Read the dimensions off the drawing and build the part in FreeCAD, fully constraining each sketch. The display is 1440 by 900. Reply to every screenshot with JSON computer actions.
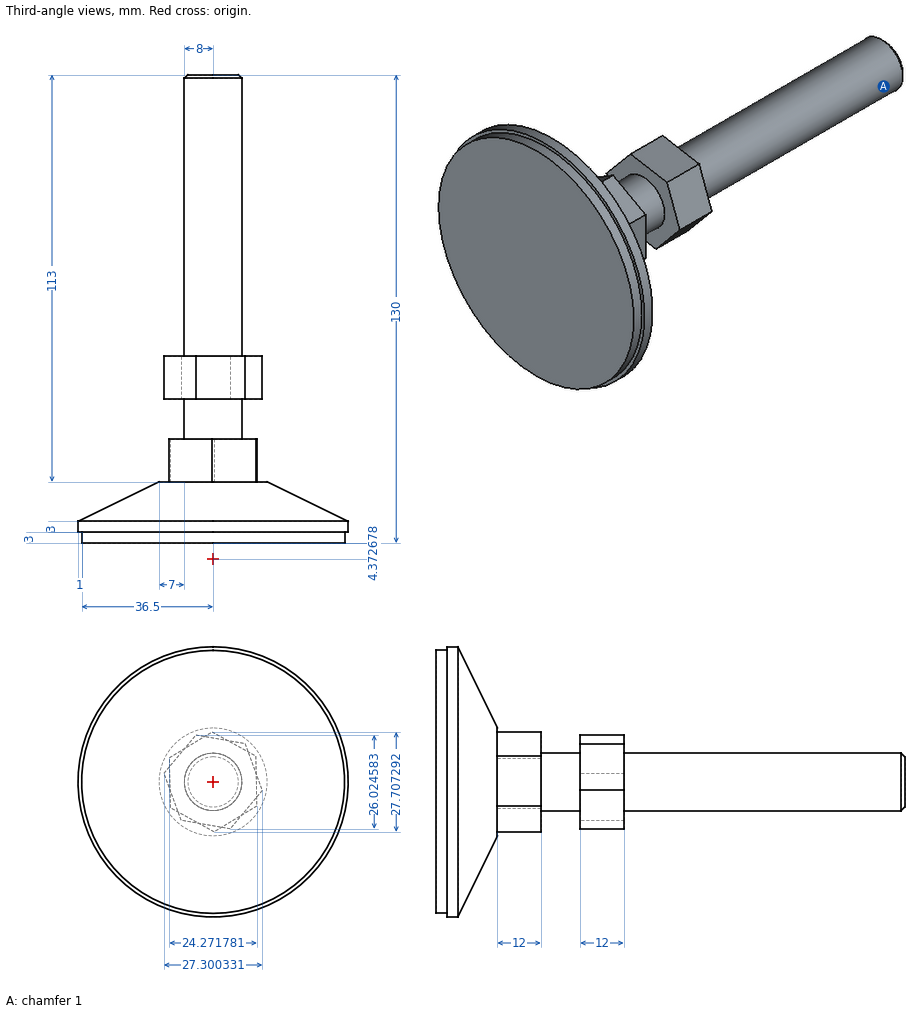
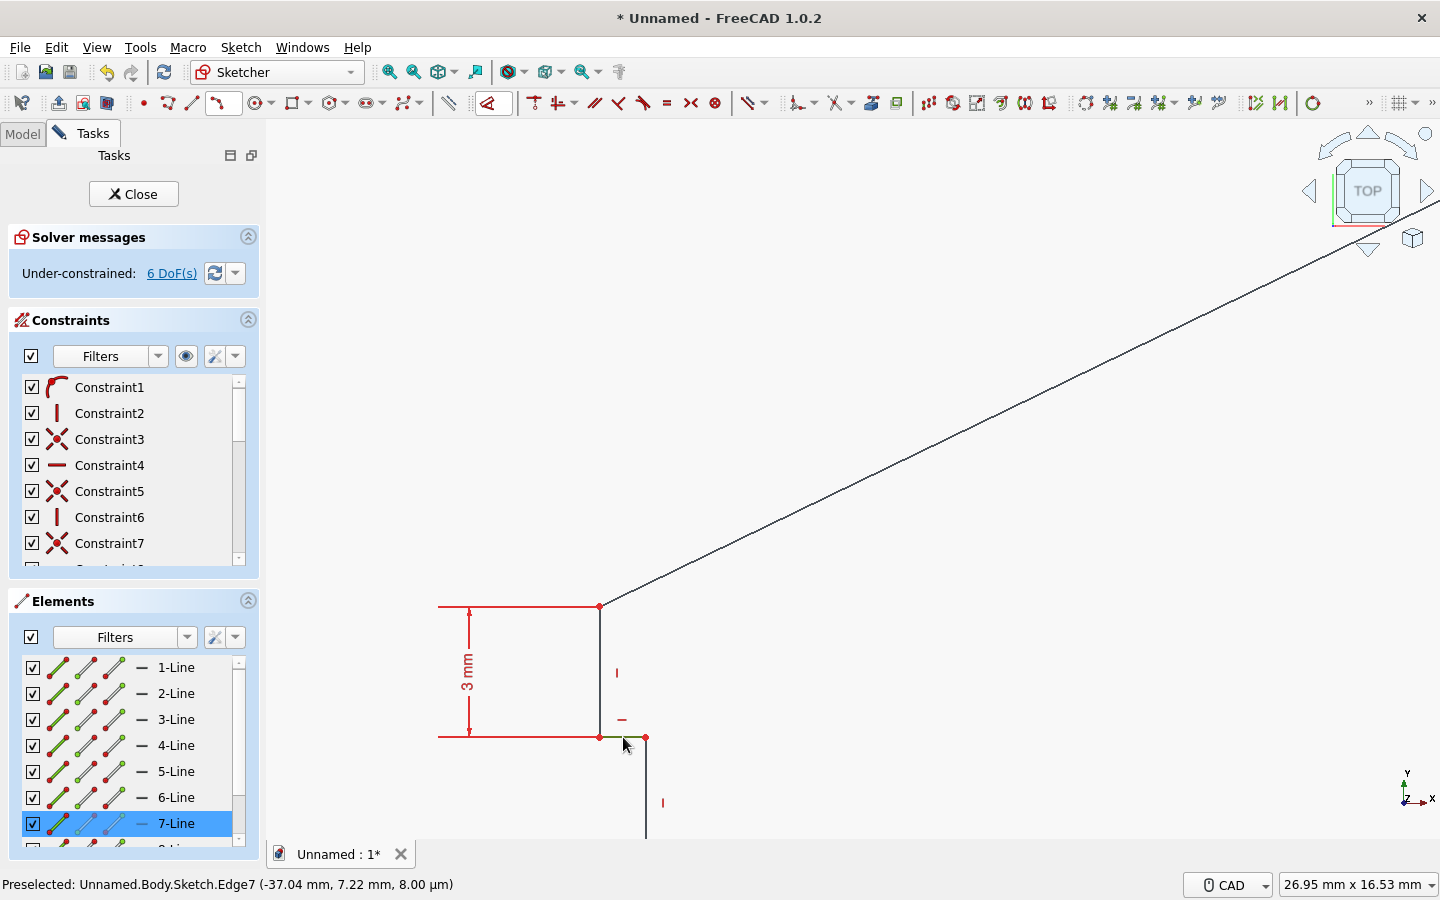
{"action": "left_click", "coordinate": [506, 104]}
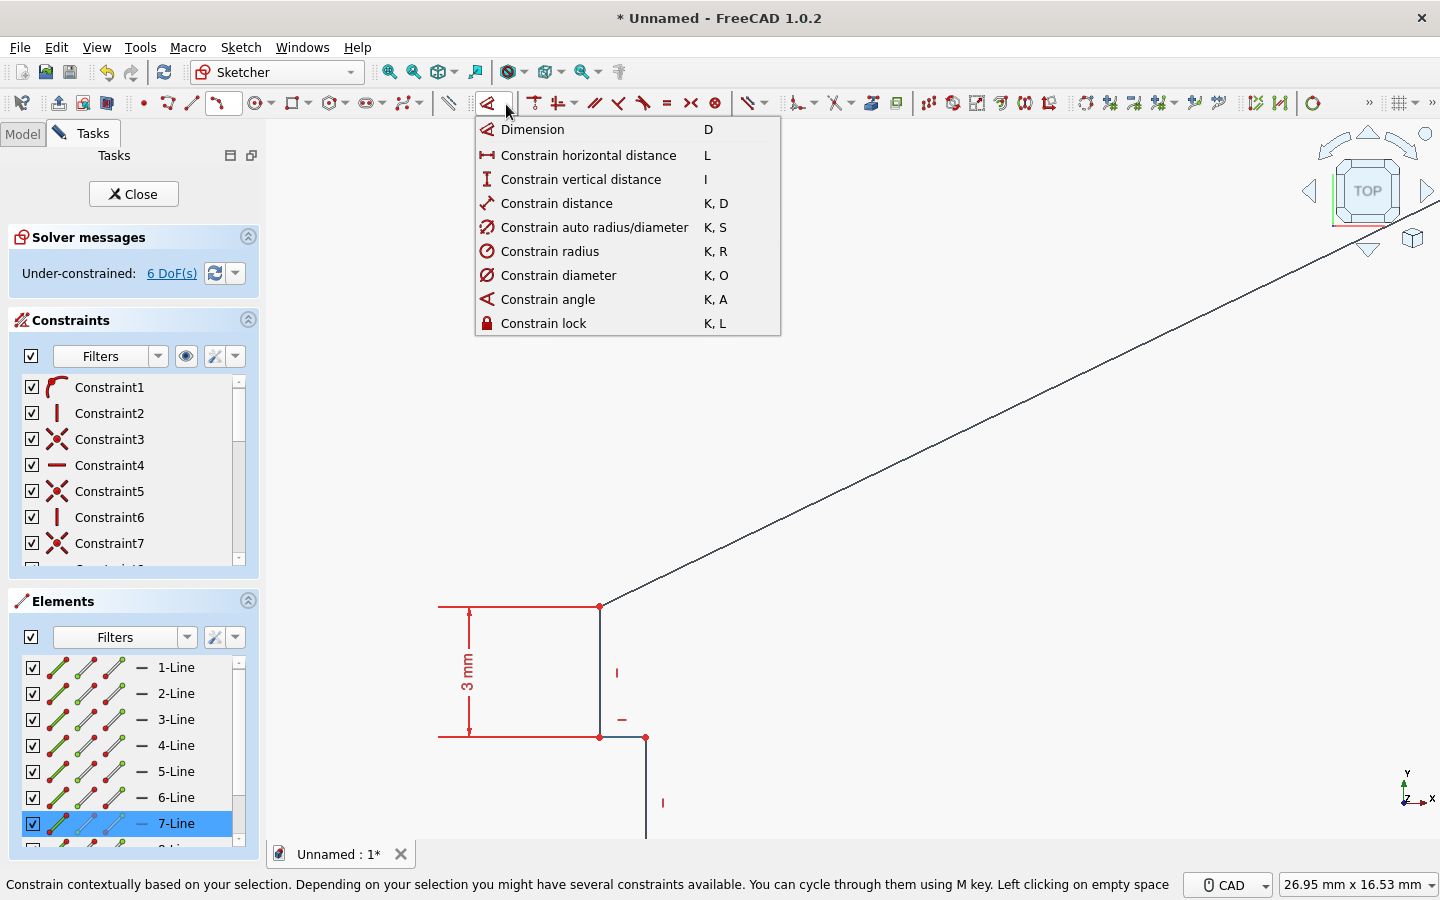
{"action": "left_click", "coordinate": [628, 155]}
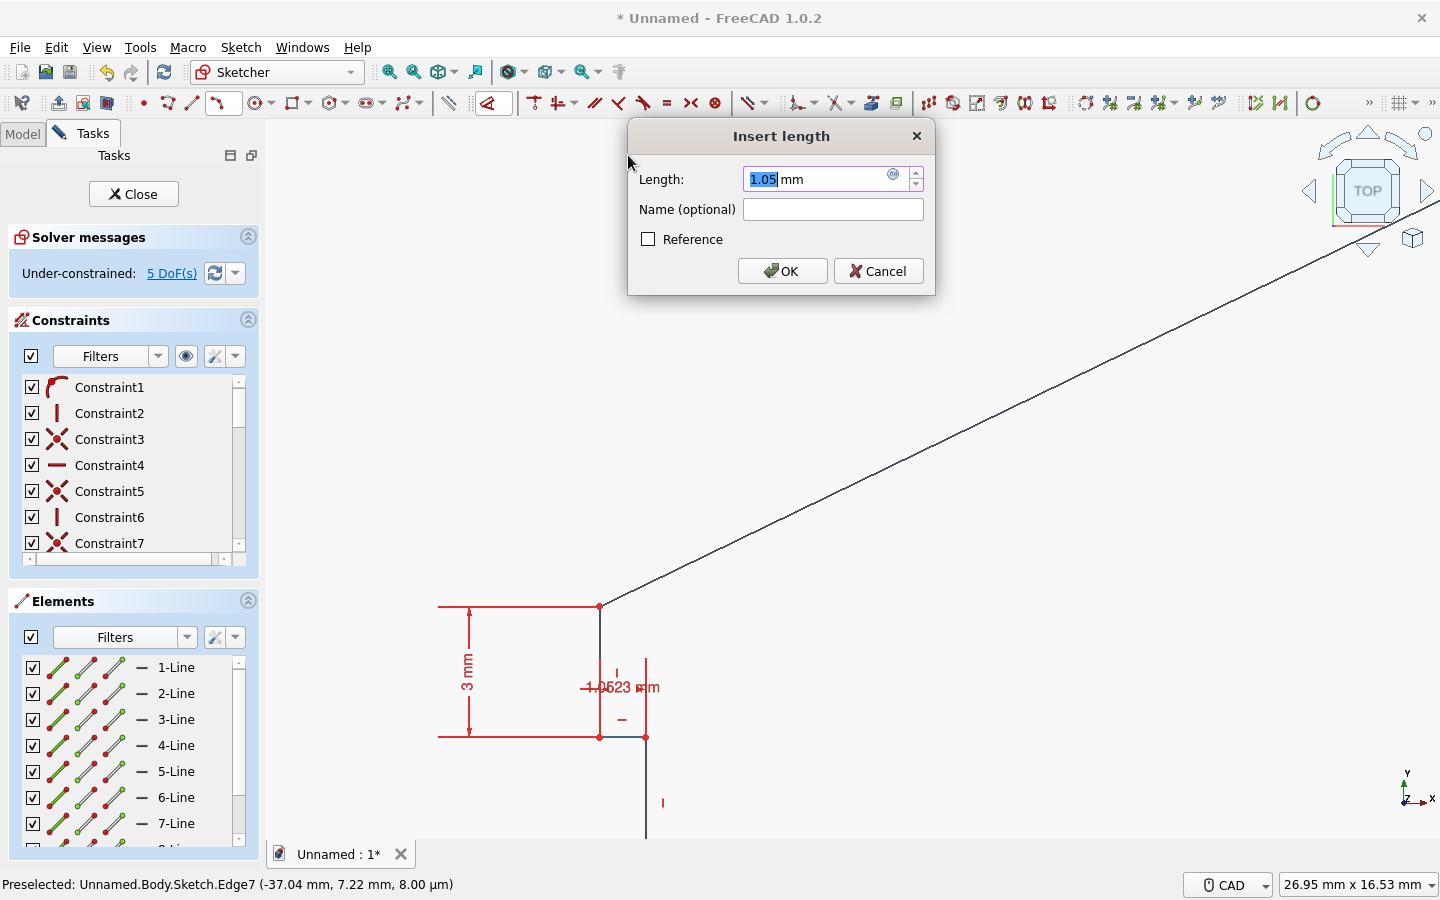
{"action": "type", "text": "1"}
{"action": "key", "text": "Return"}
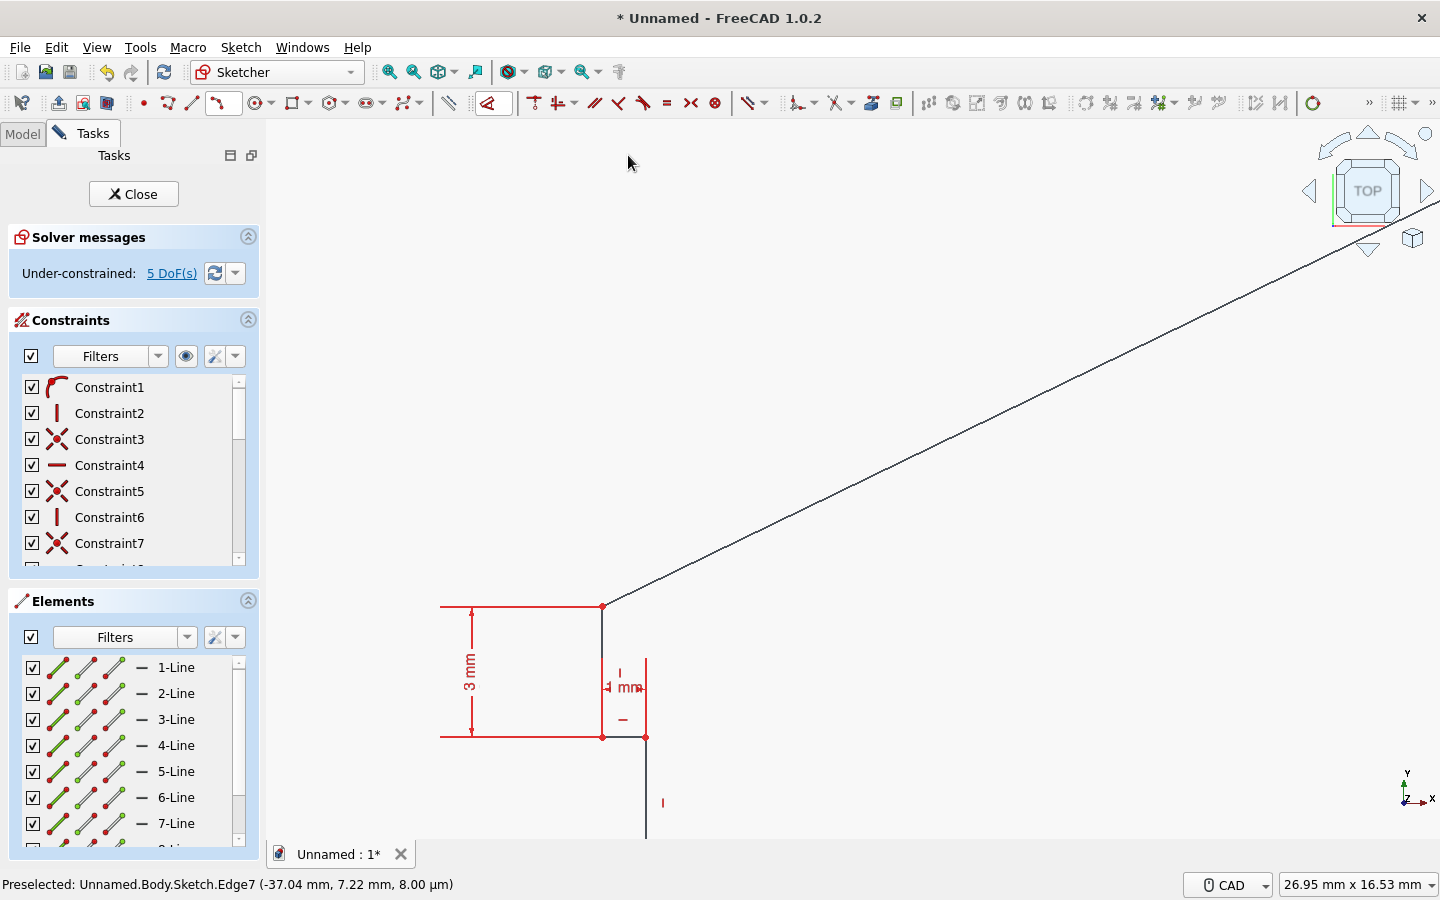
{"action": "left_click", "coordinate": [646, 776]}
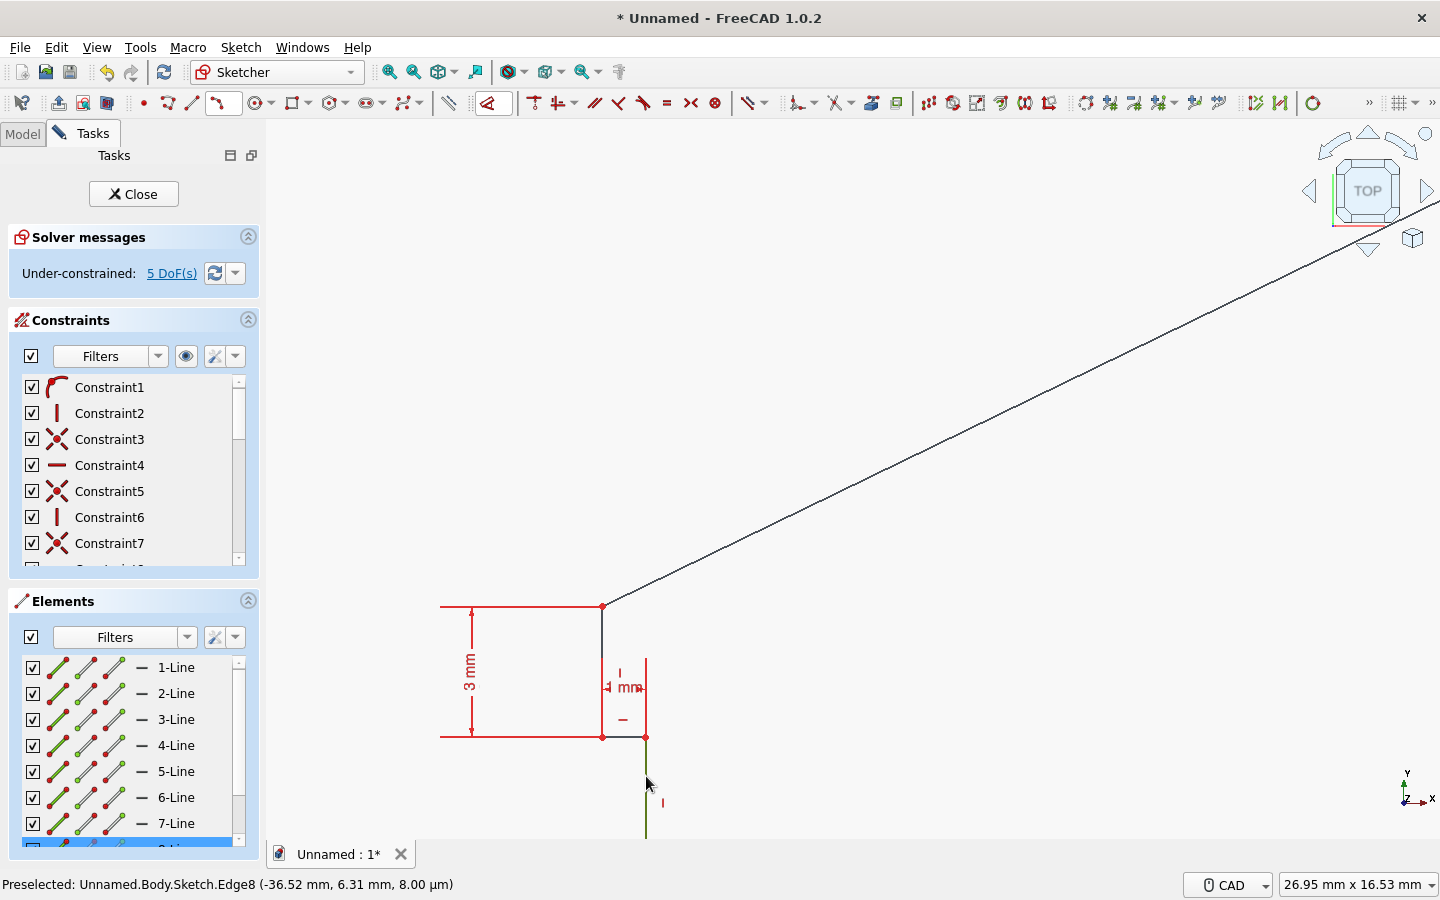
{"action": "left_click", "coordinate": [506, 104]}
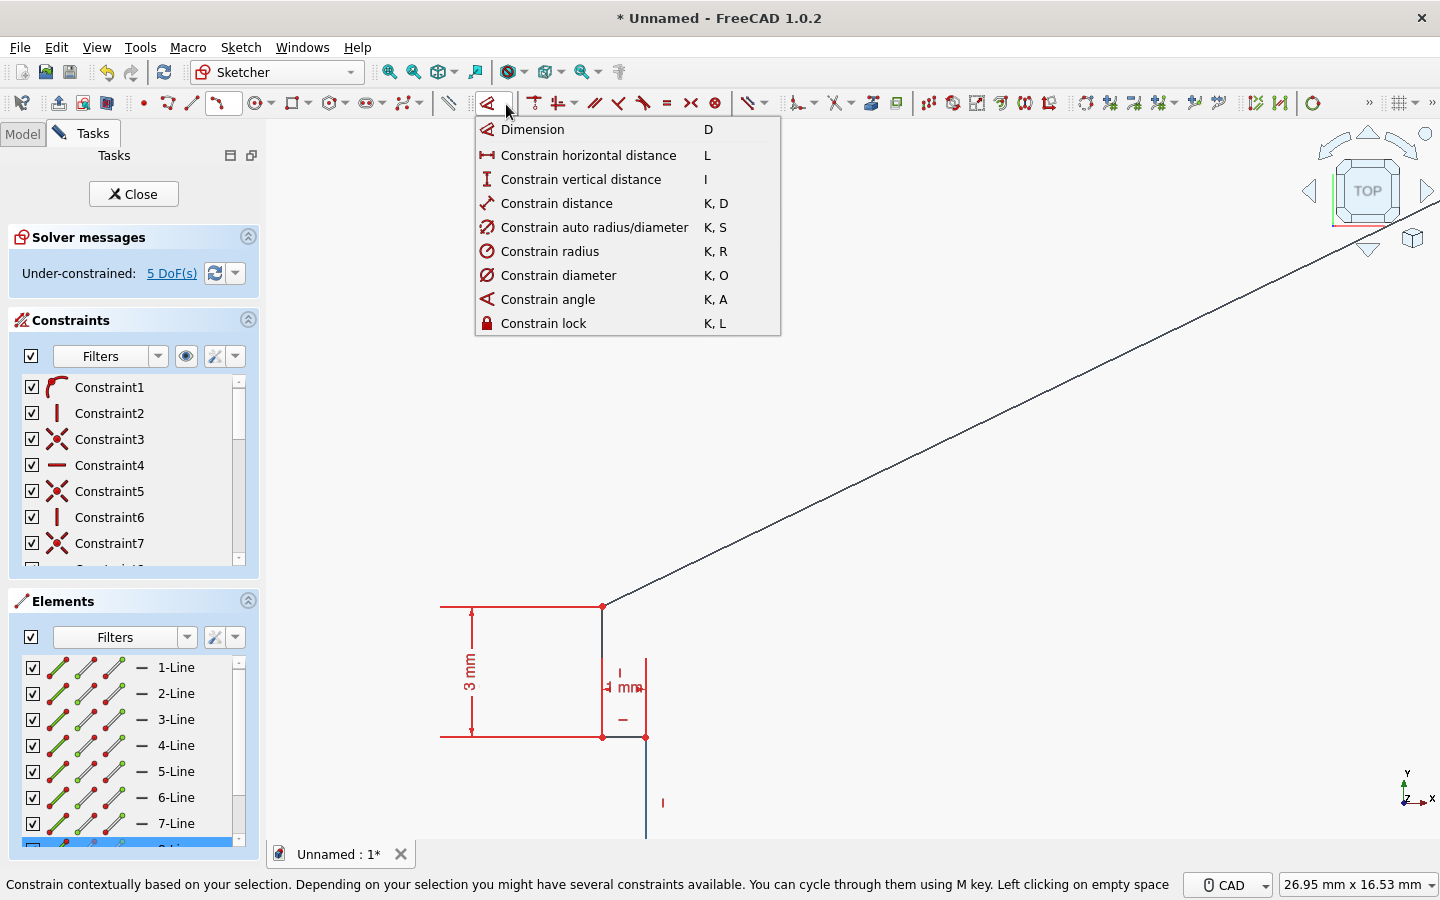
{"action": "left_click", "coordinate": [628, 179]}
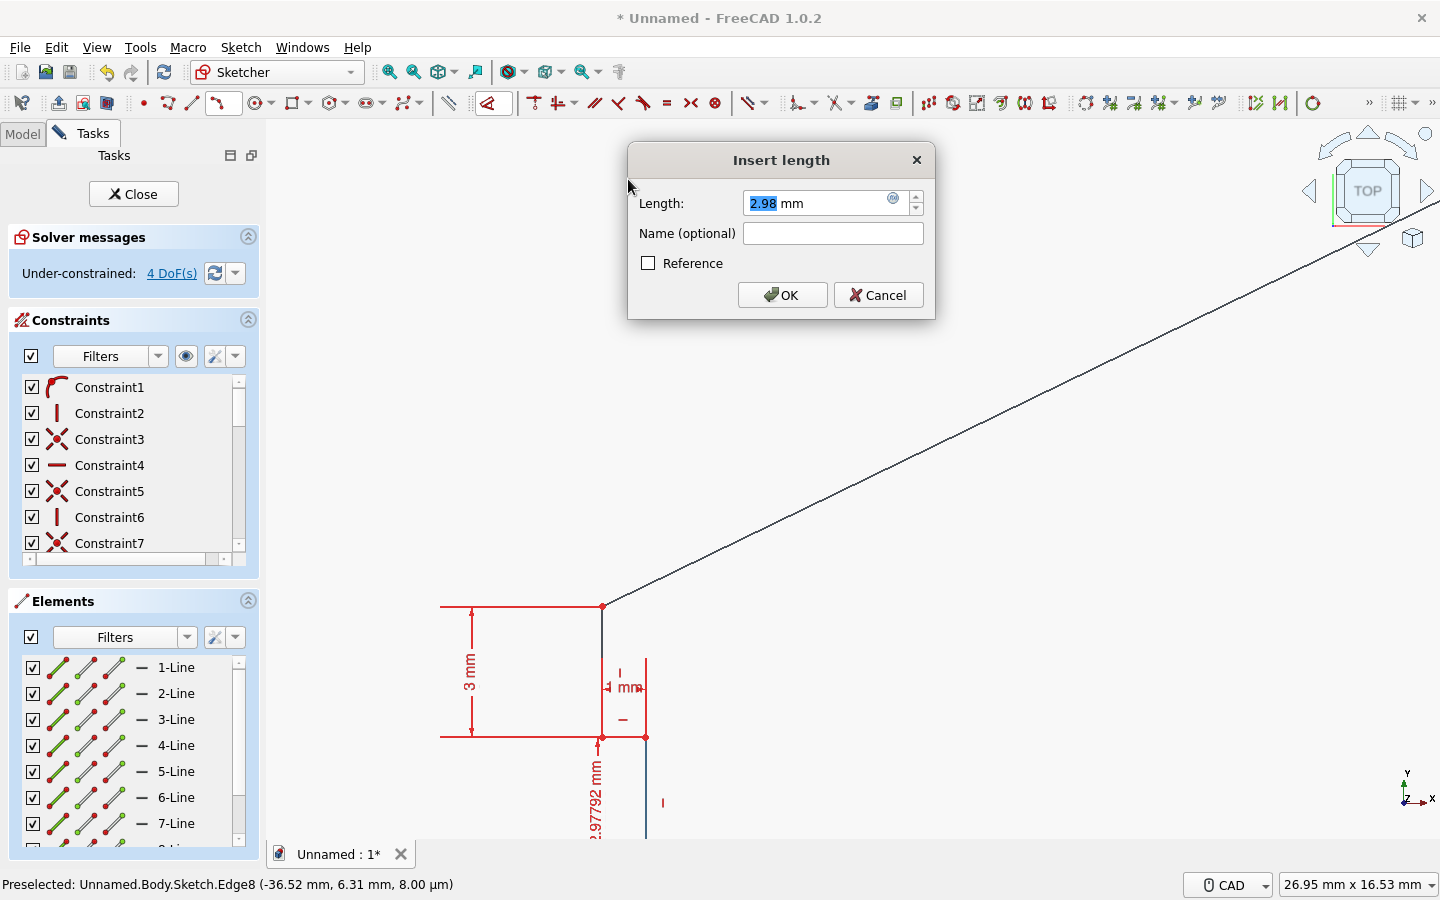
{"action": "type", "text": "3"}
{"action": "key", "text": "Return"}